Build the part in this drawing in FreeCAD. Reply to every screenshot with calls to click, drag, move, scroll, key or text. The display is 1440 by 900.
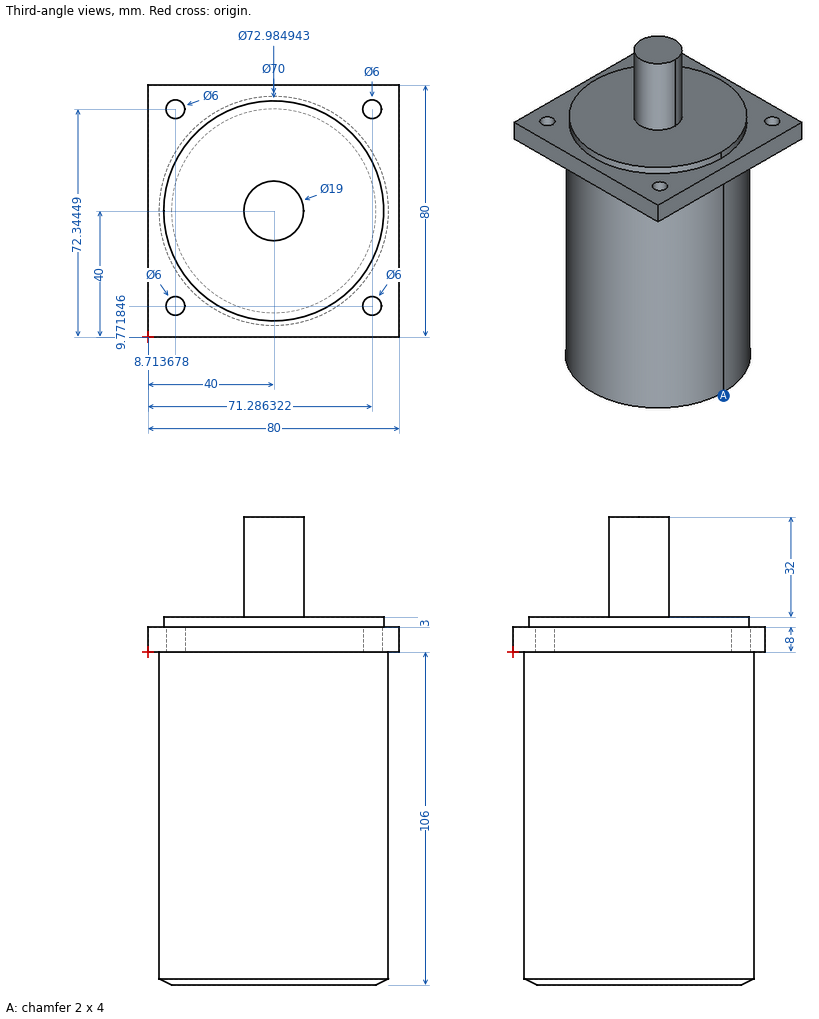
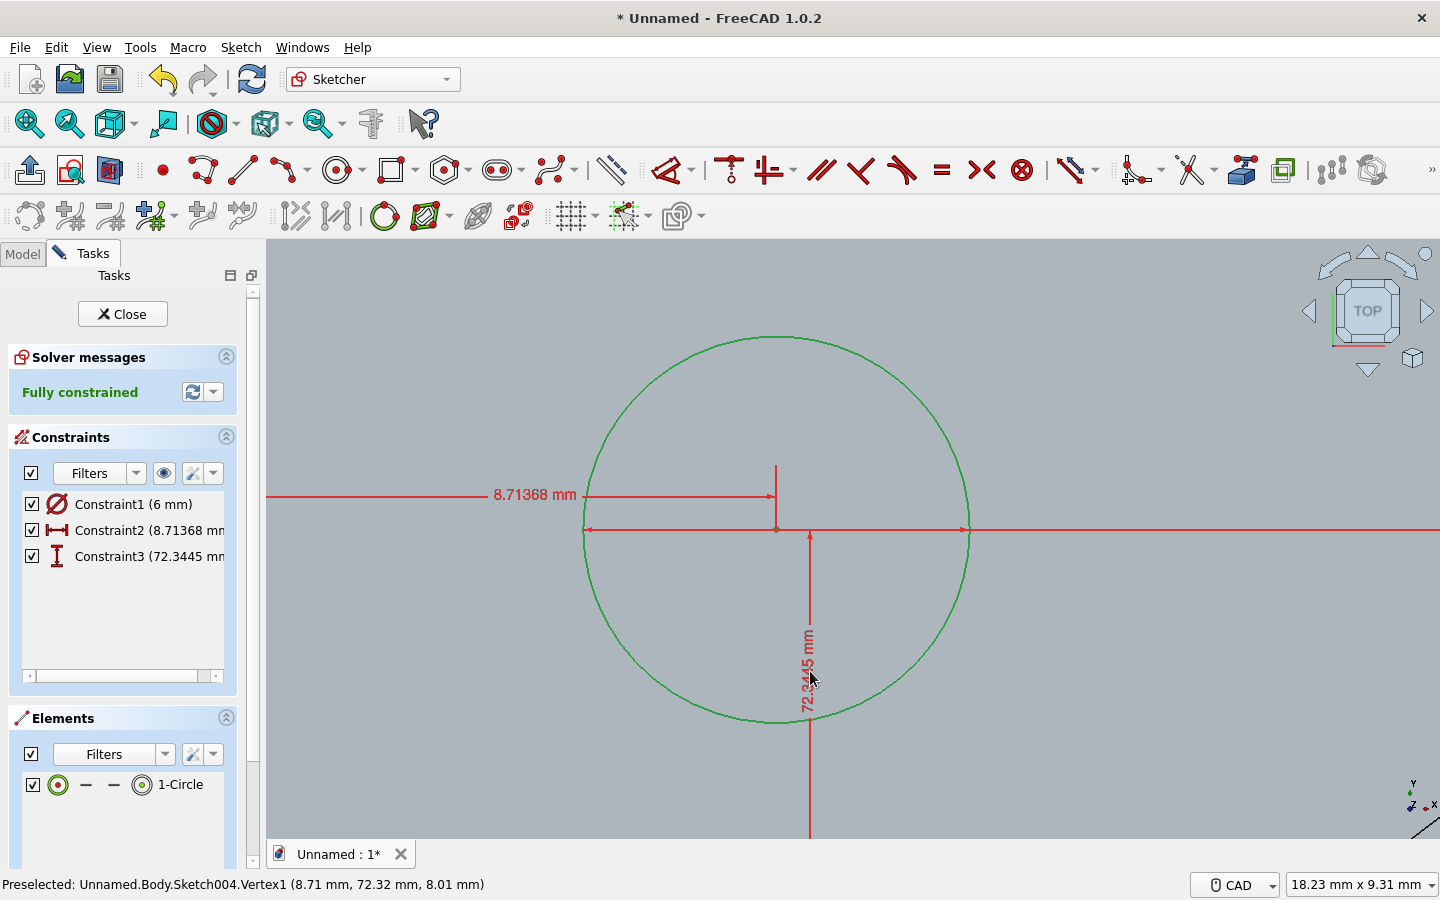
click(123, 314)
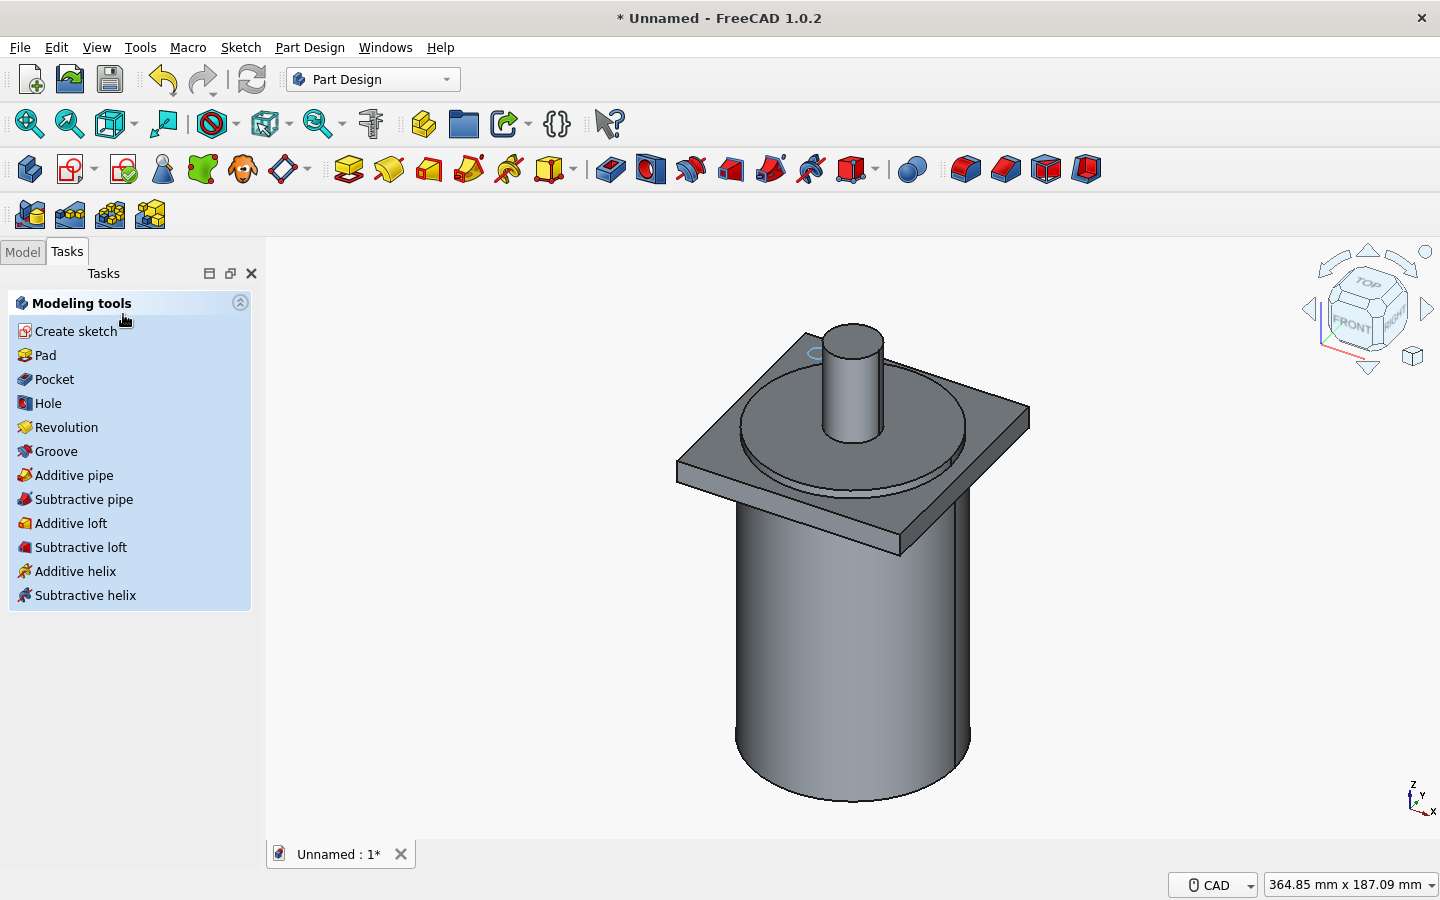
click(612, 170)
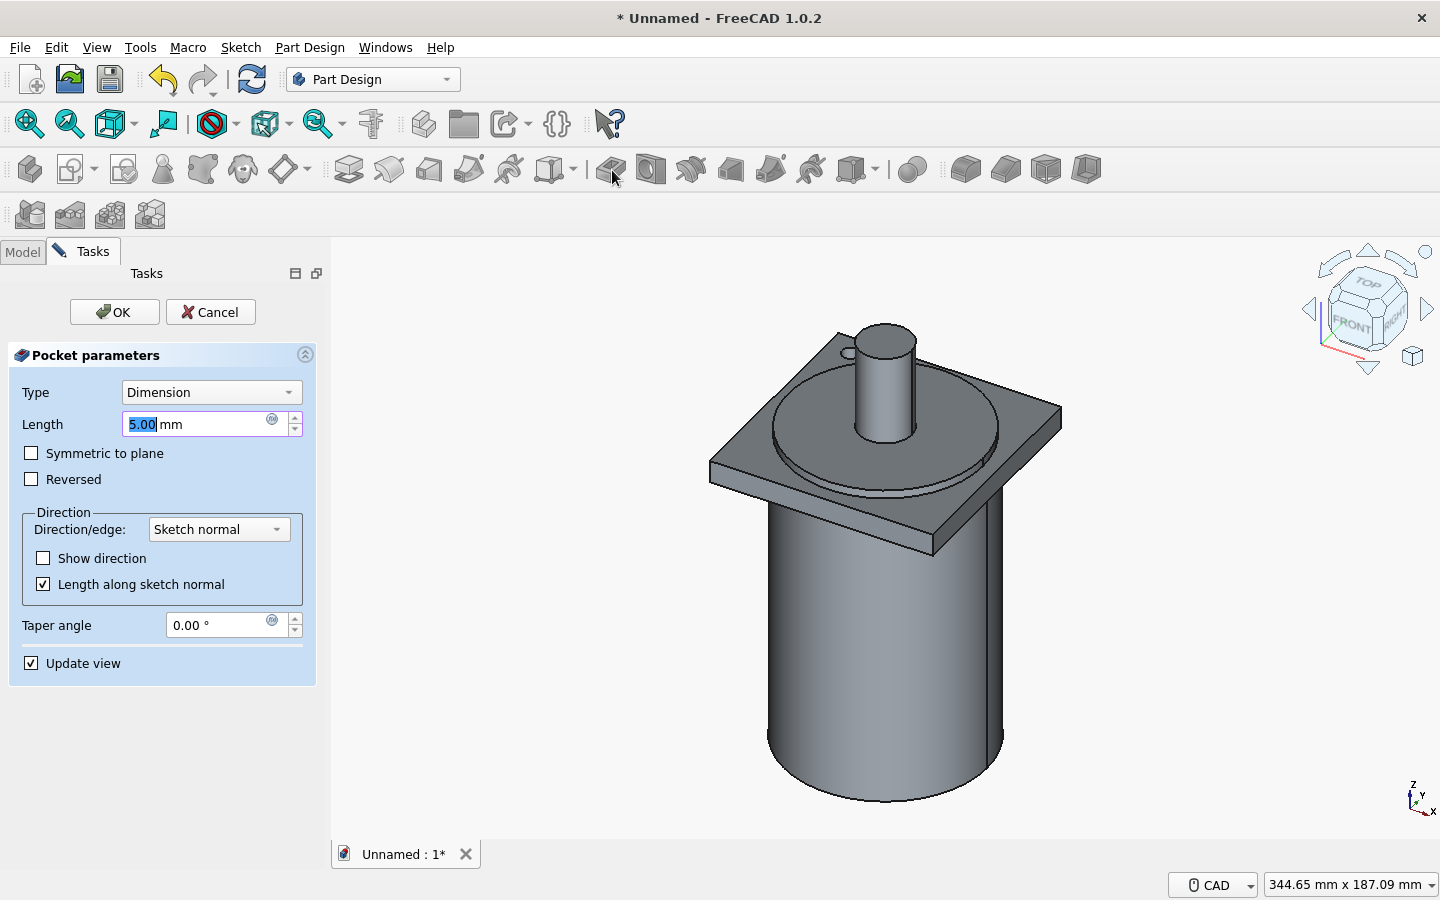
click(212, 392)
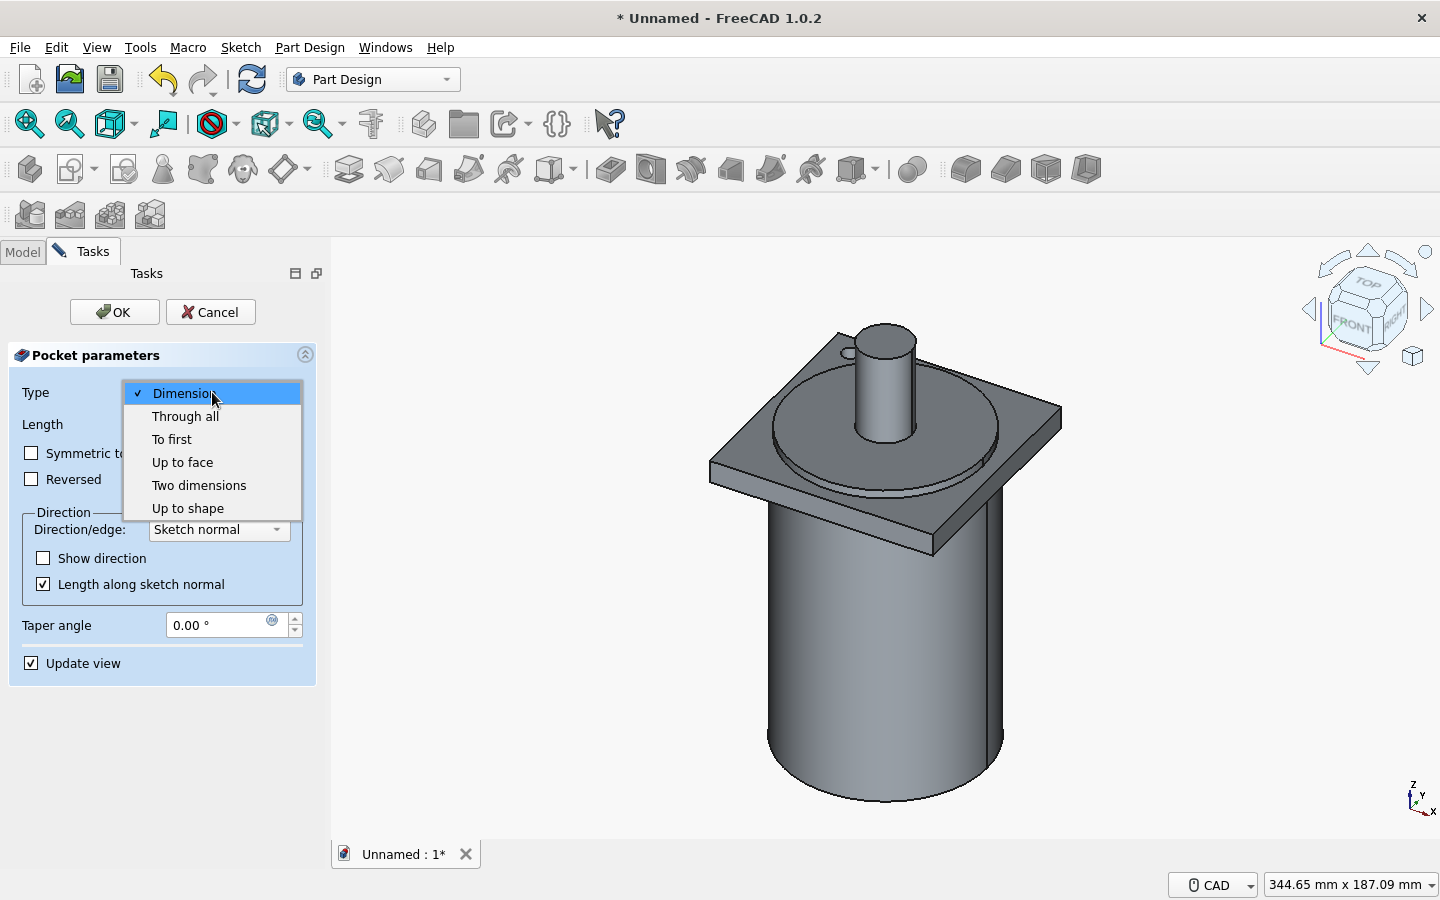
click(212, 440)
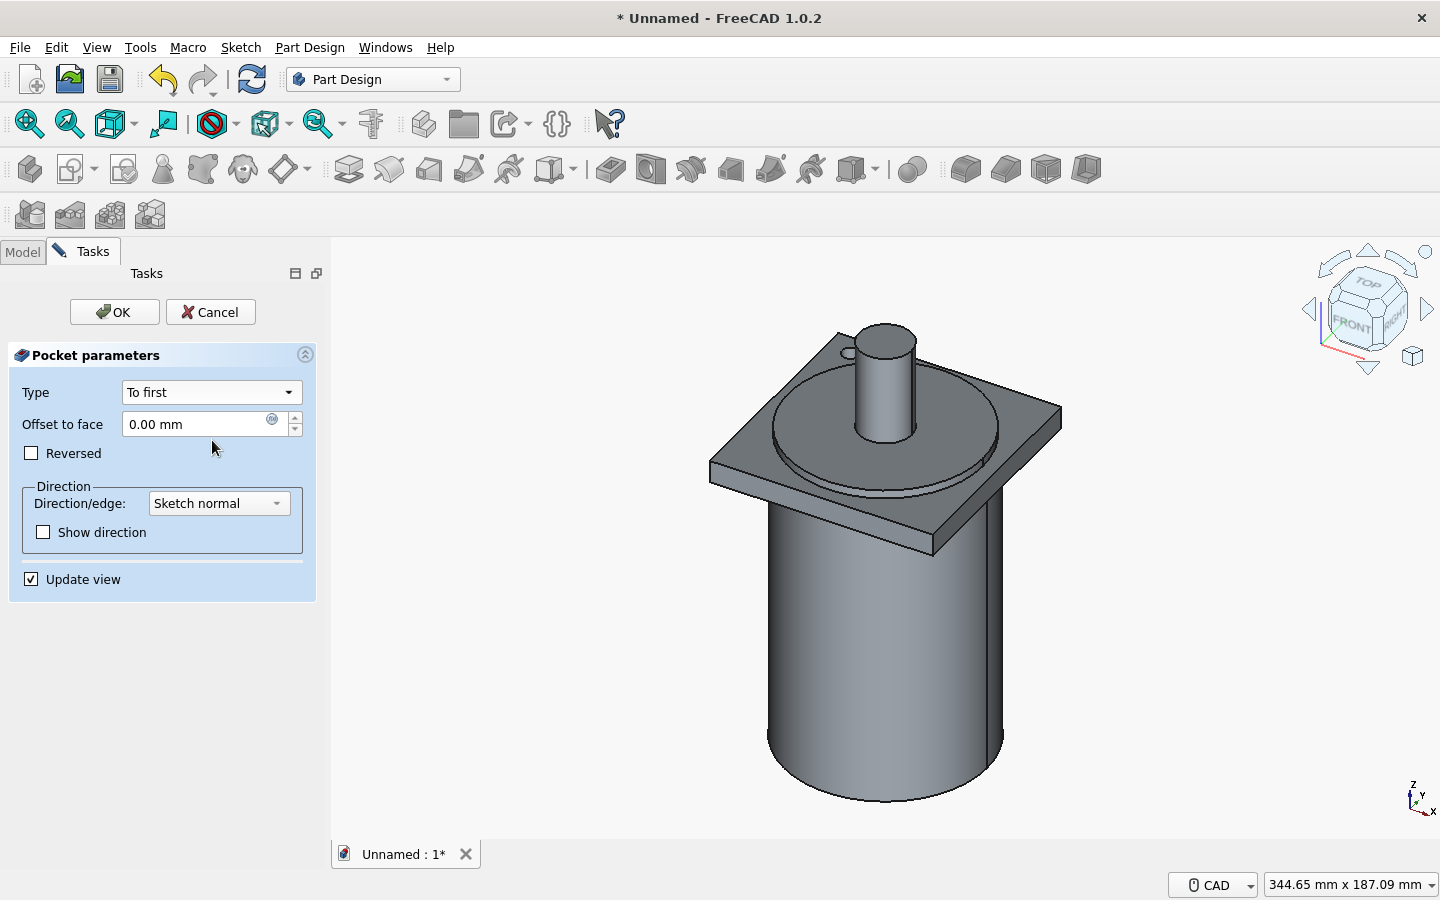
click(115, 312)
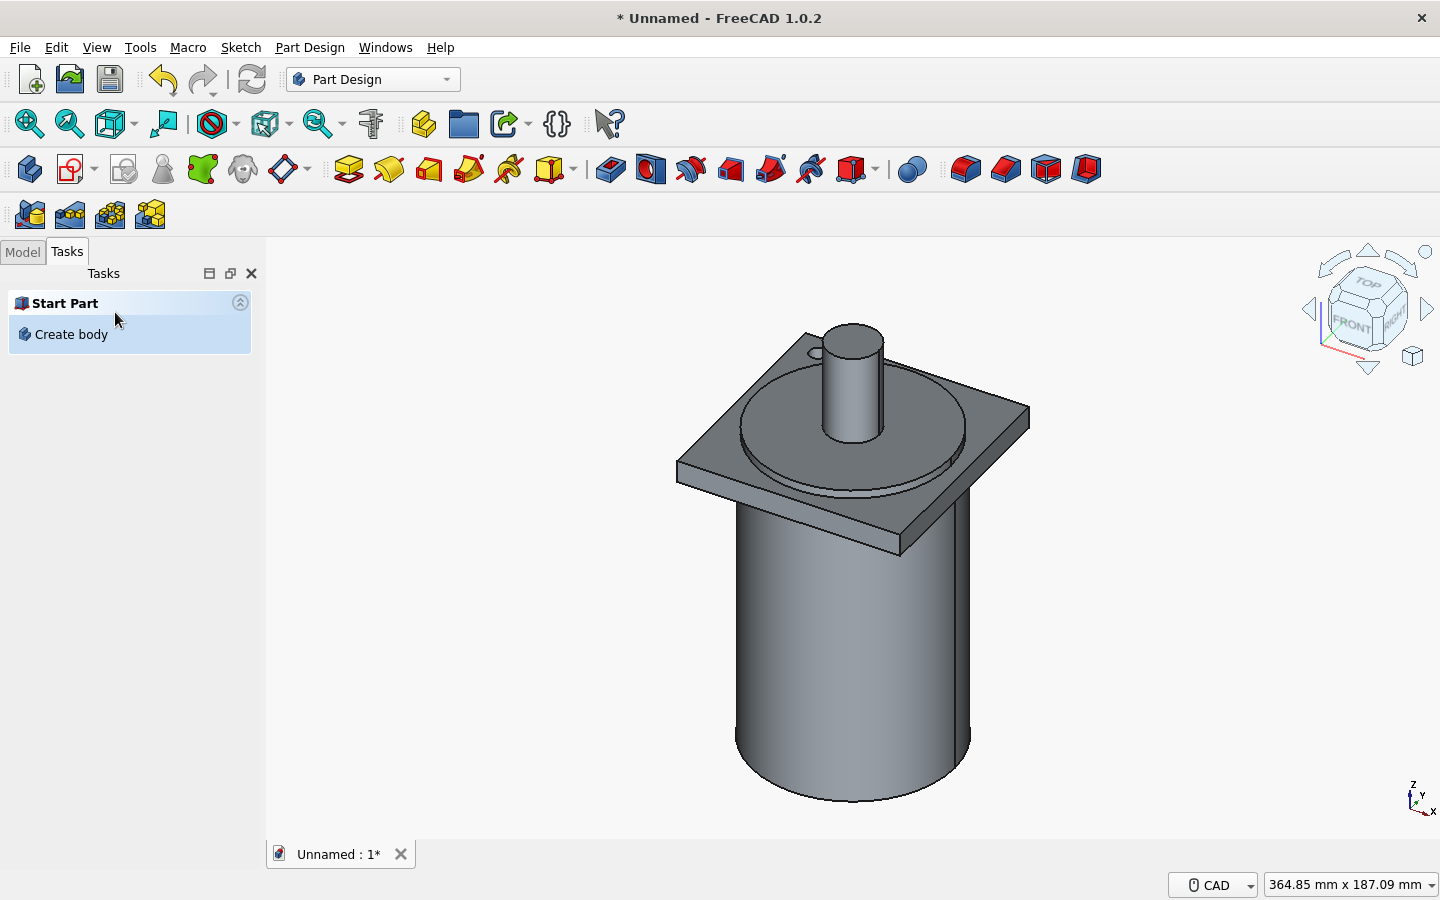
click(862, 509)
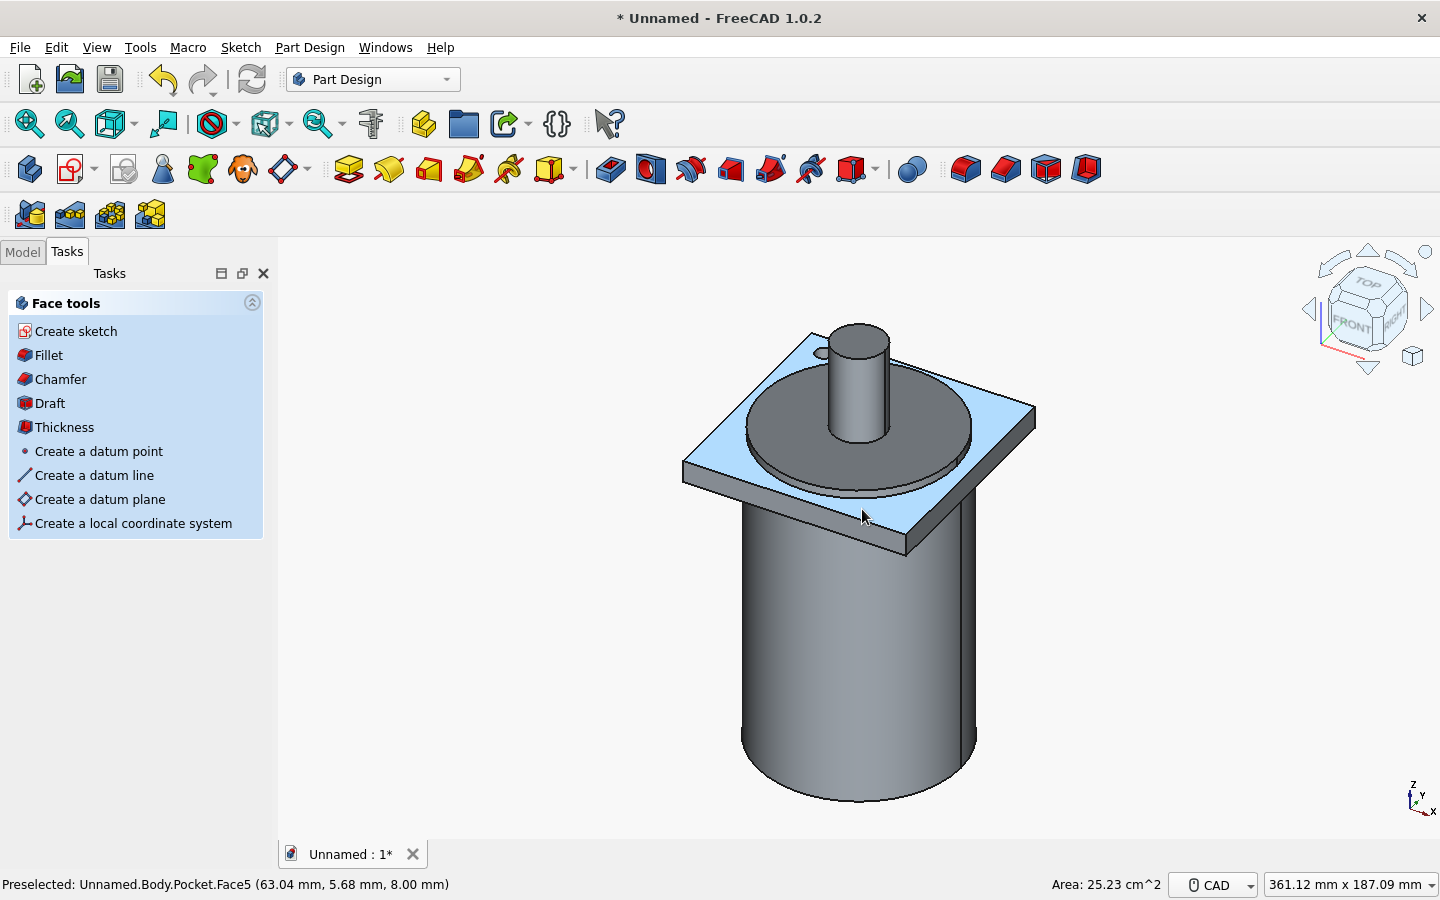
click(70, 170)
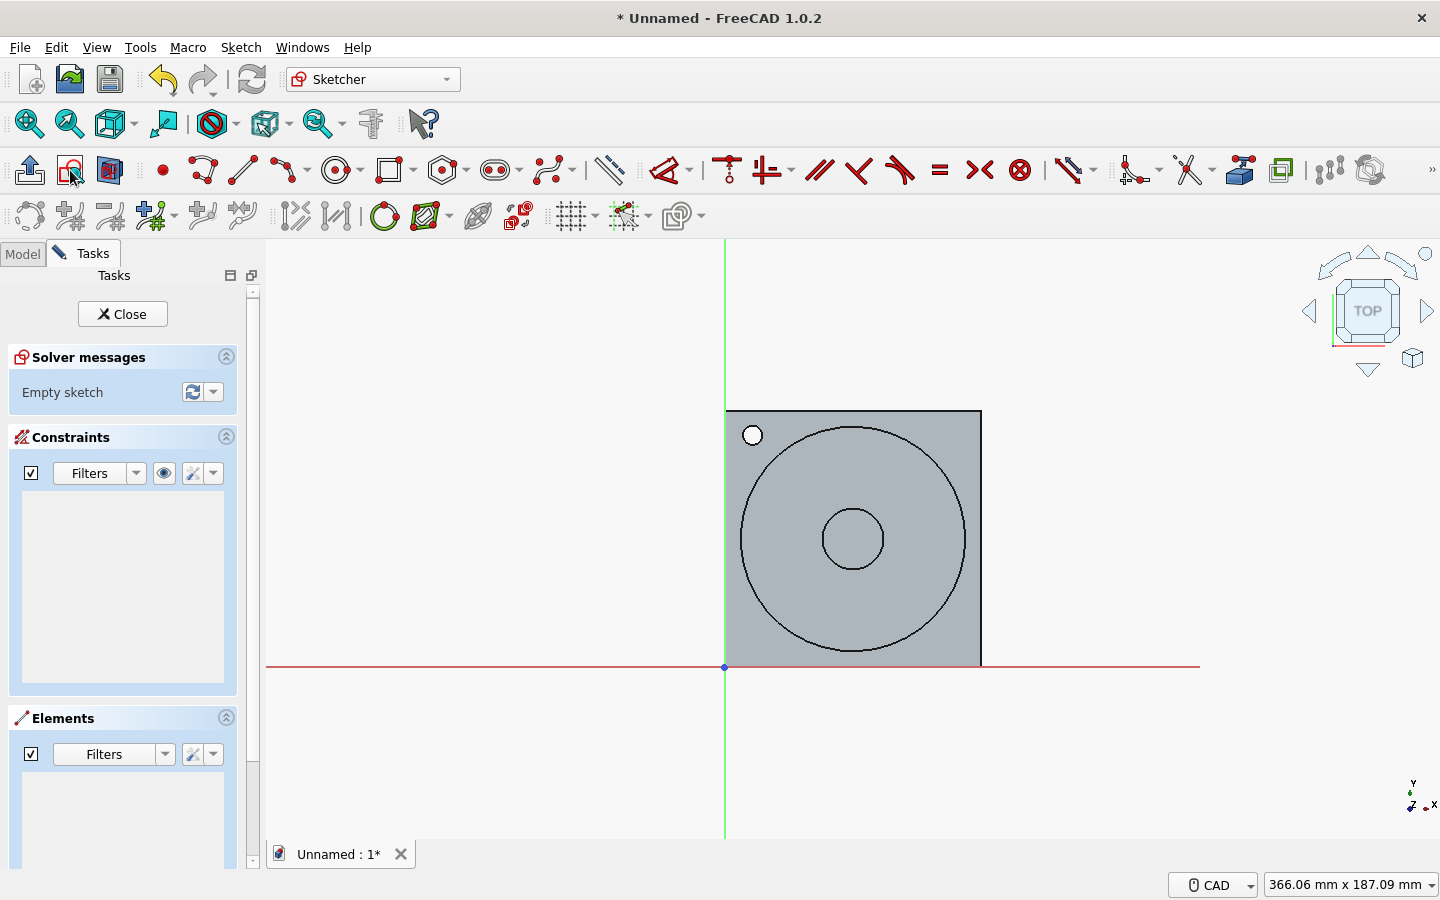
scroll(962, 430, up, 15)